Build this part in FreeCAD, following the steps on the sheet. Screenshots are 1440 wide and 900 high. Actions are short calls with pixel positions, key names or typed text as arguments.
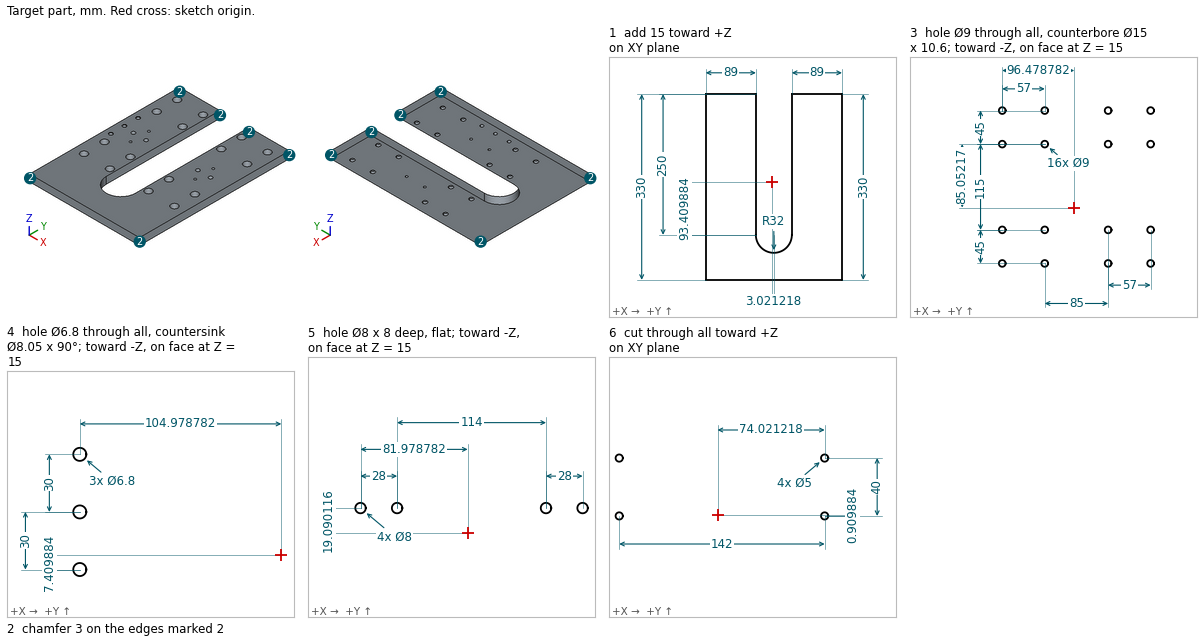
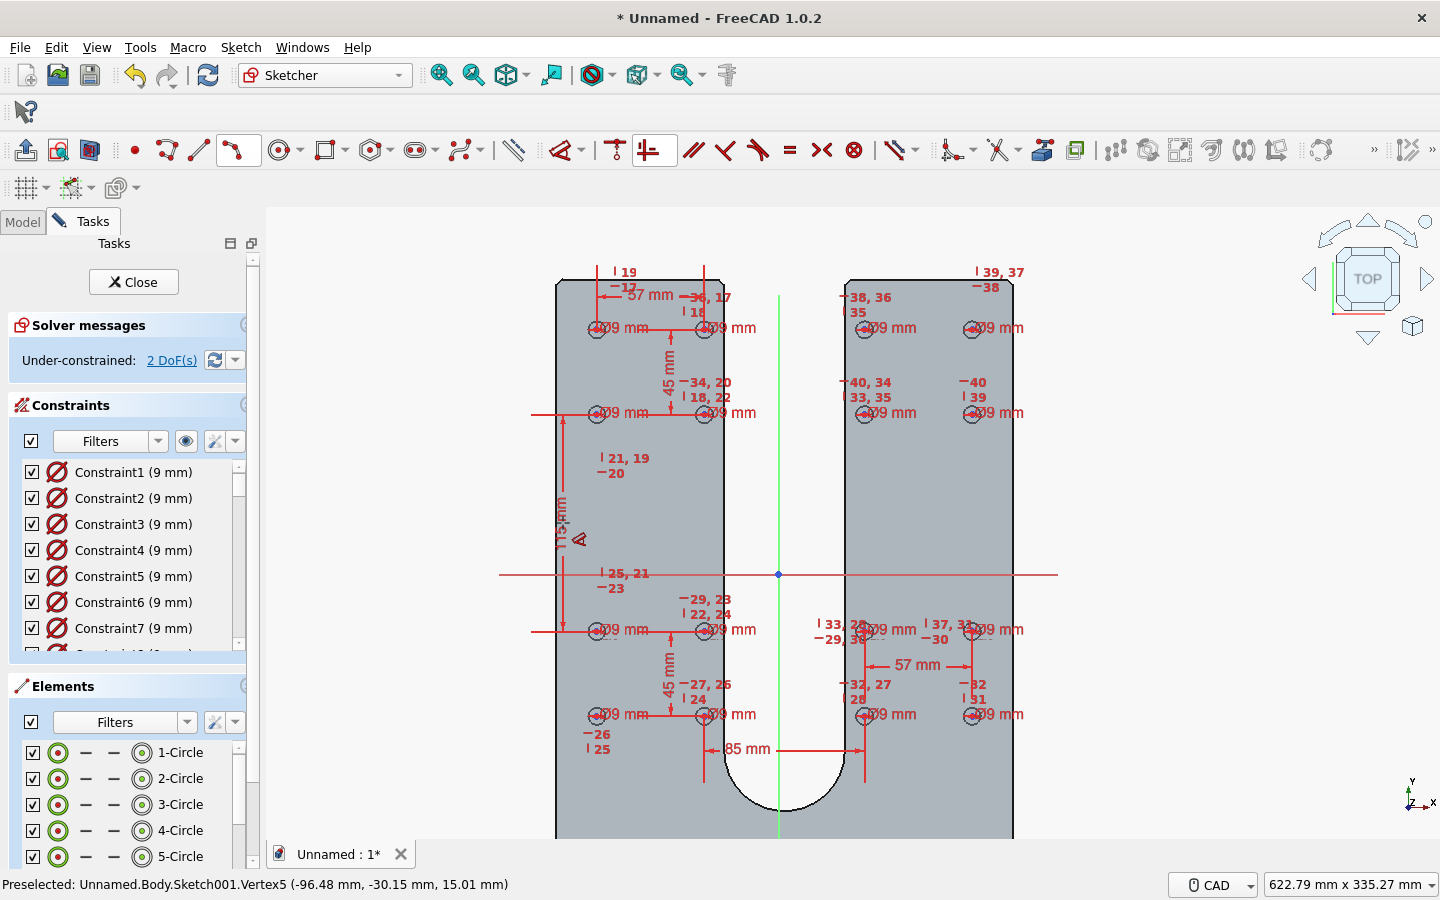
click(704, 415)
click(670, 495)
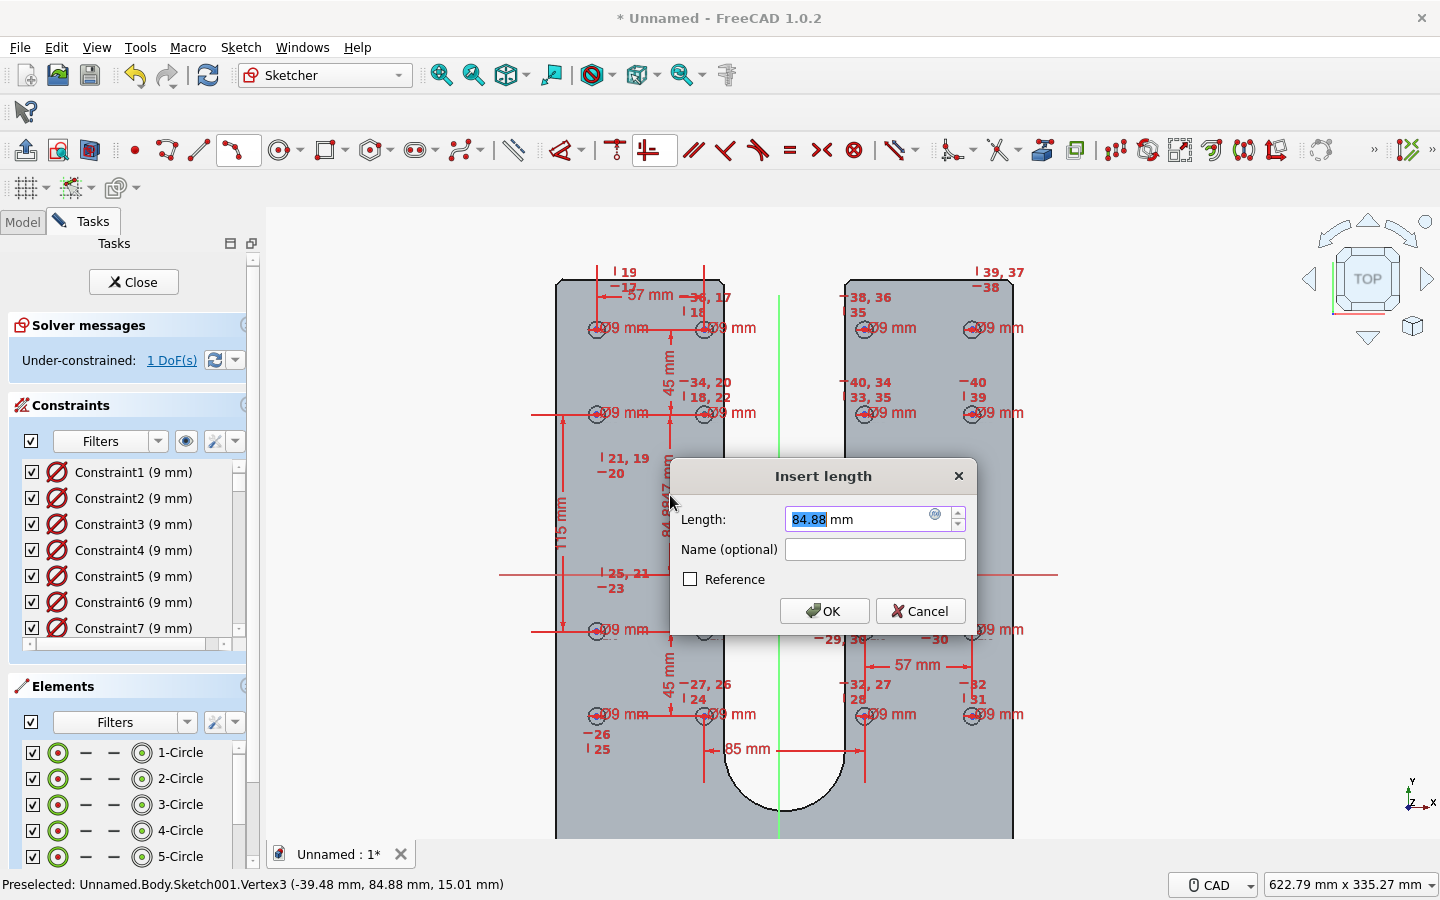
text(85.05217)
key(Return)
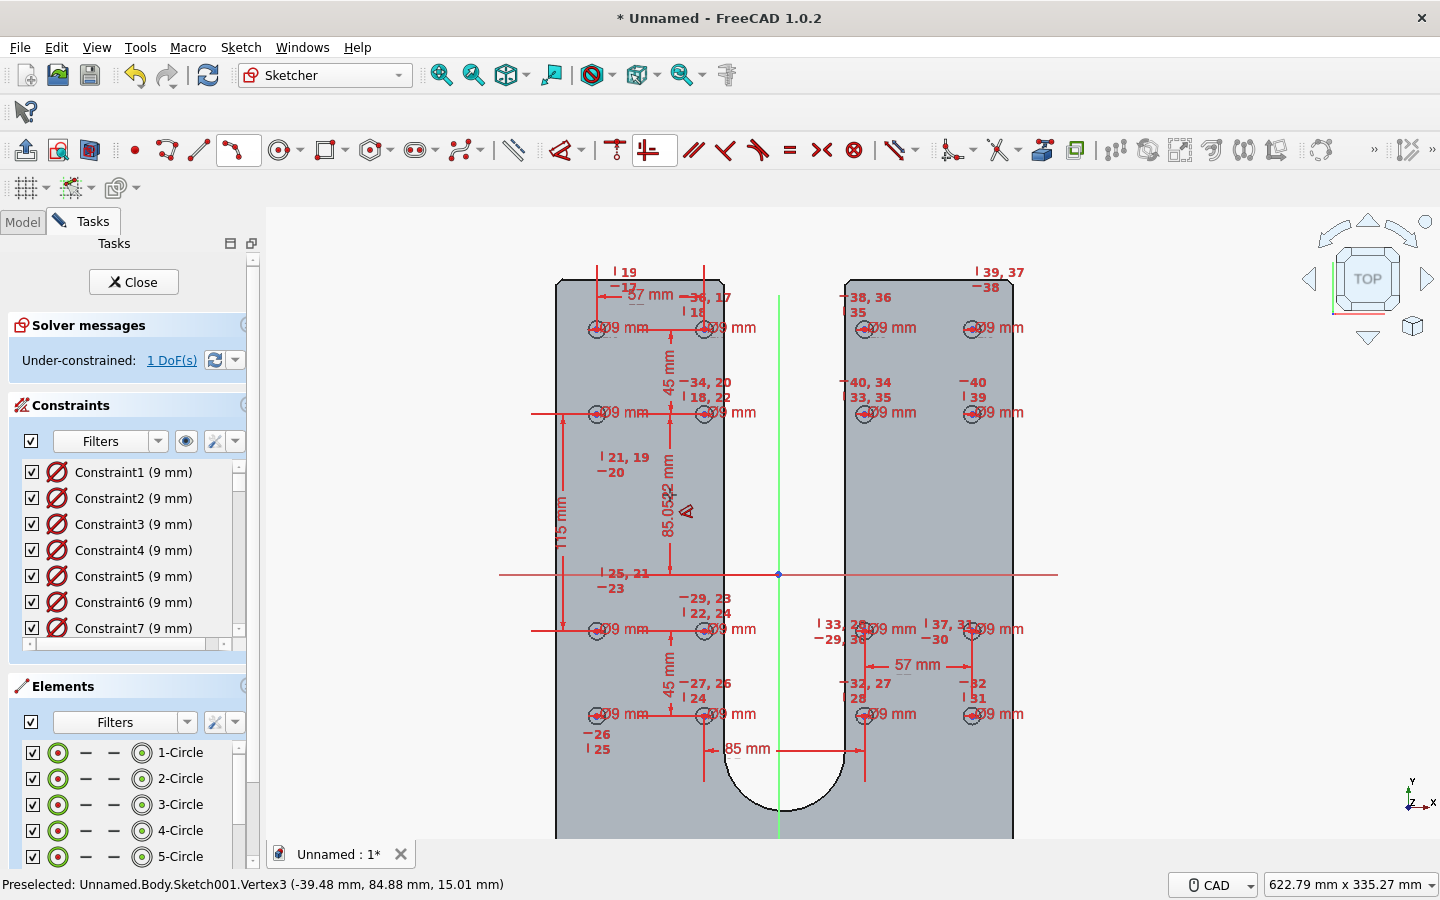
click(597, 330)
click(730, 296)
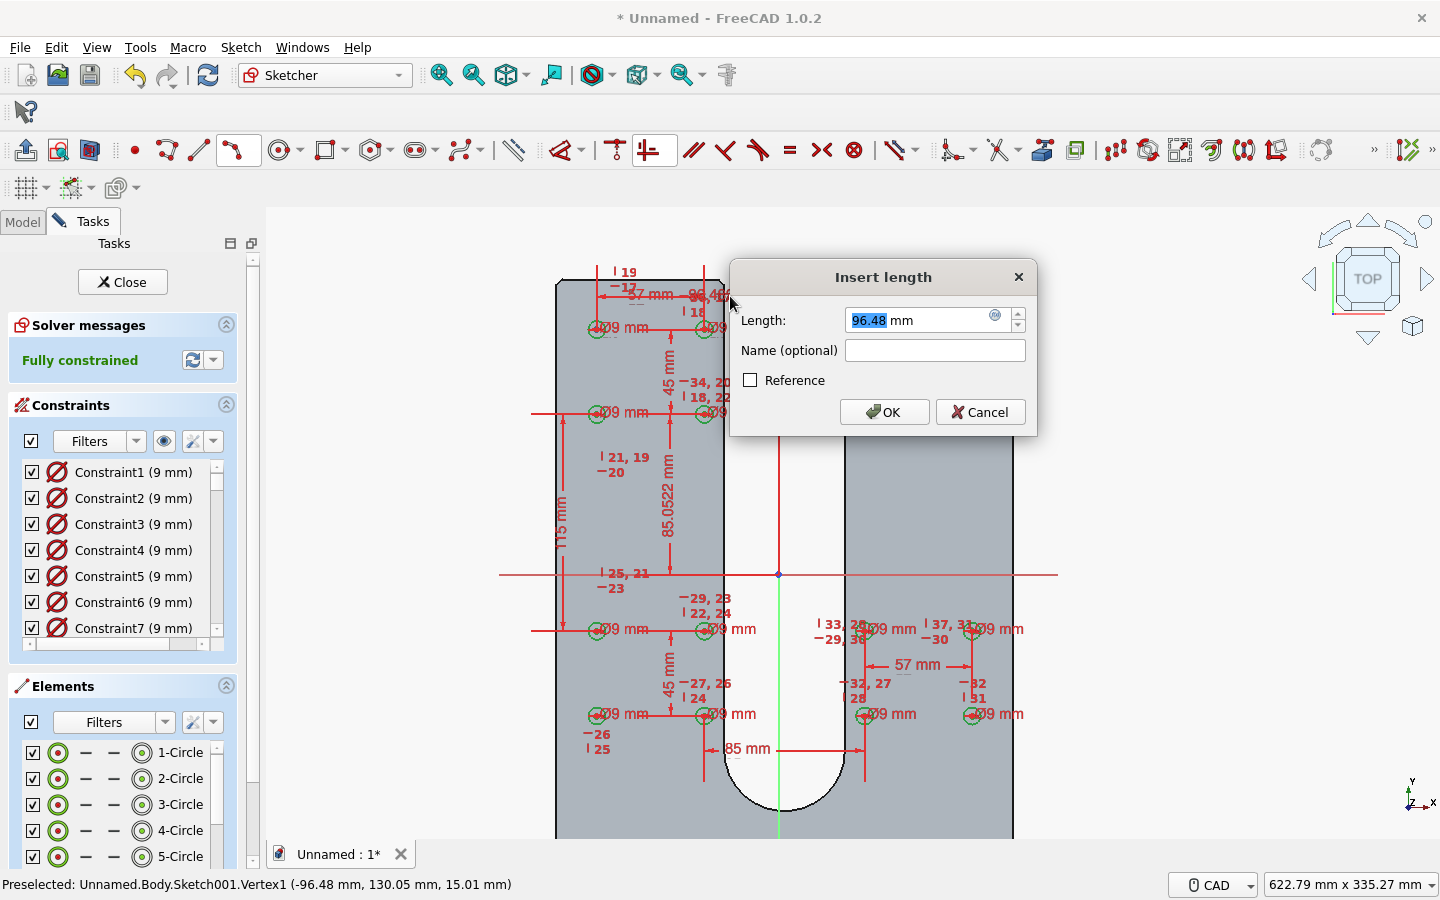
text(96.478782)
key(Return)
key(Escape)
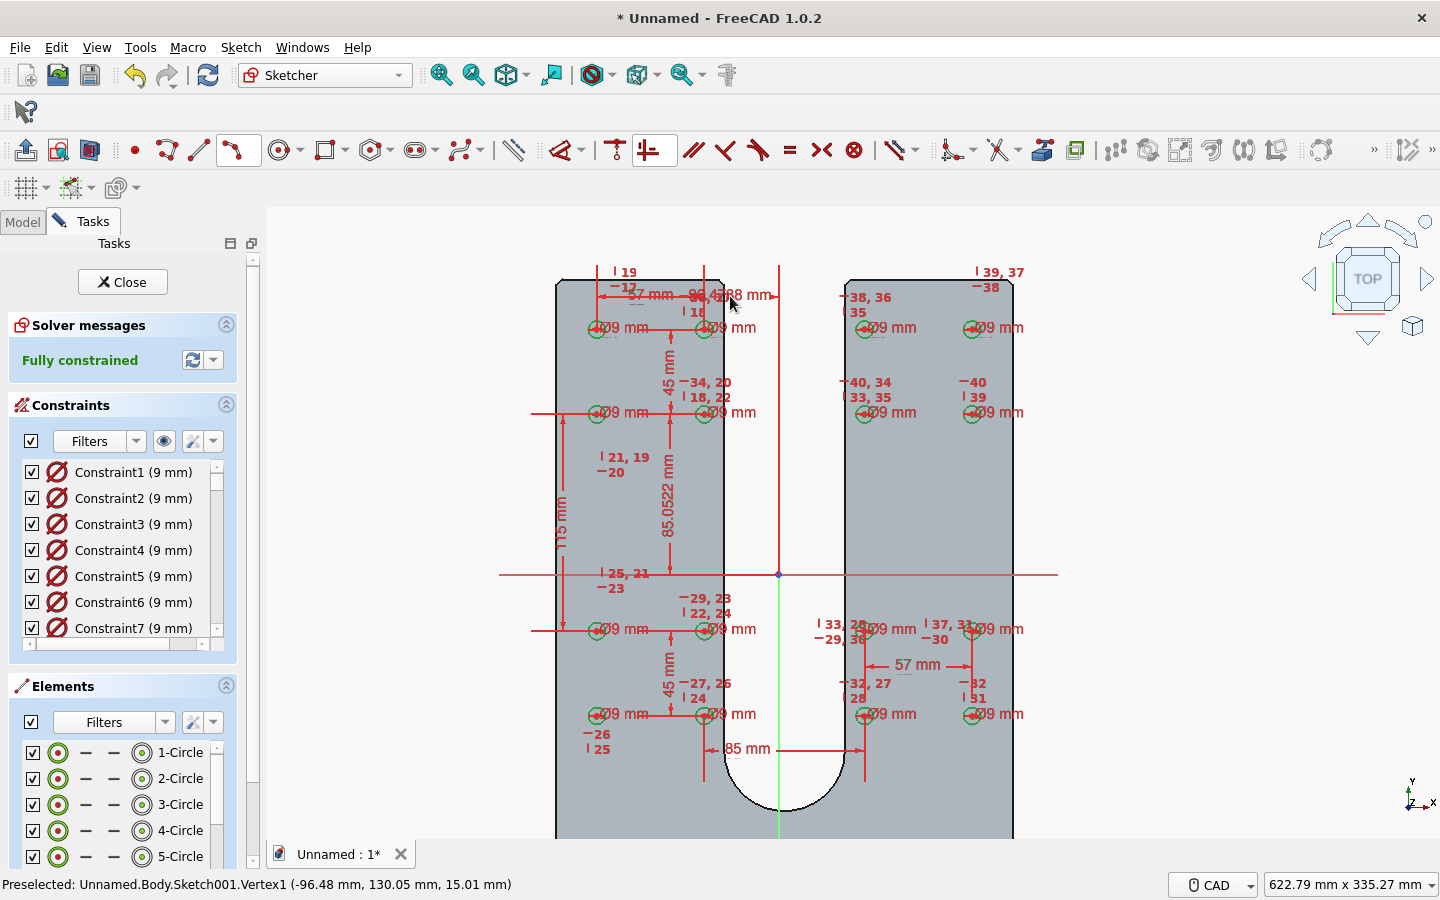
click(123, 282)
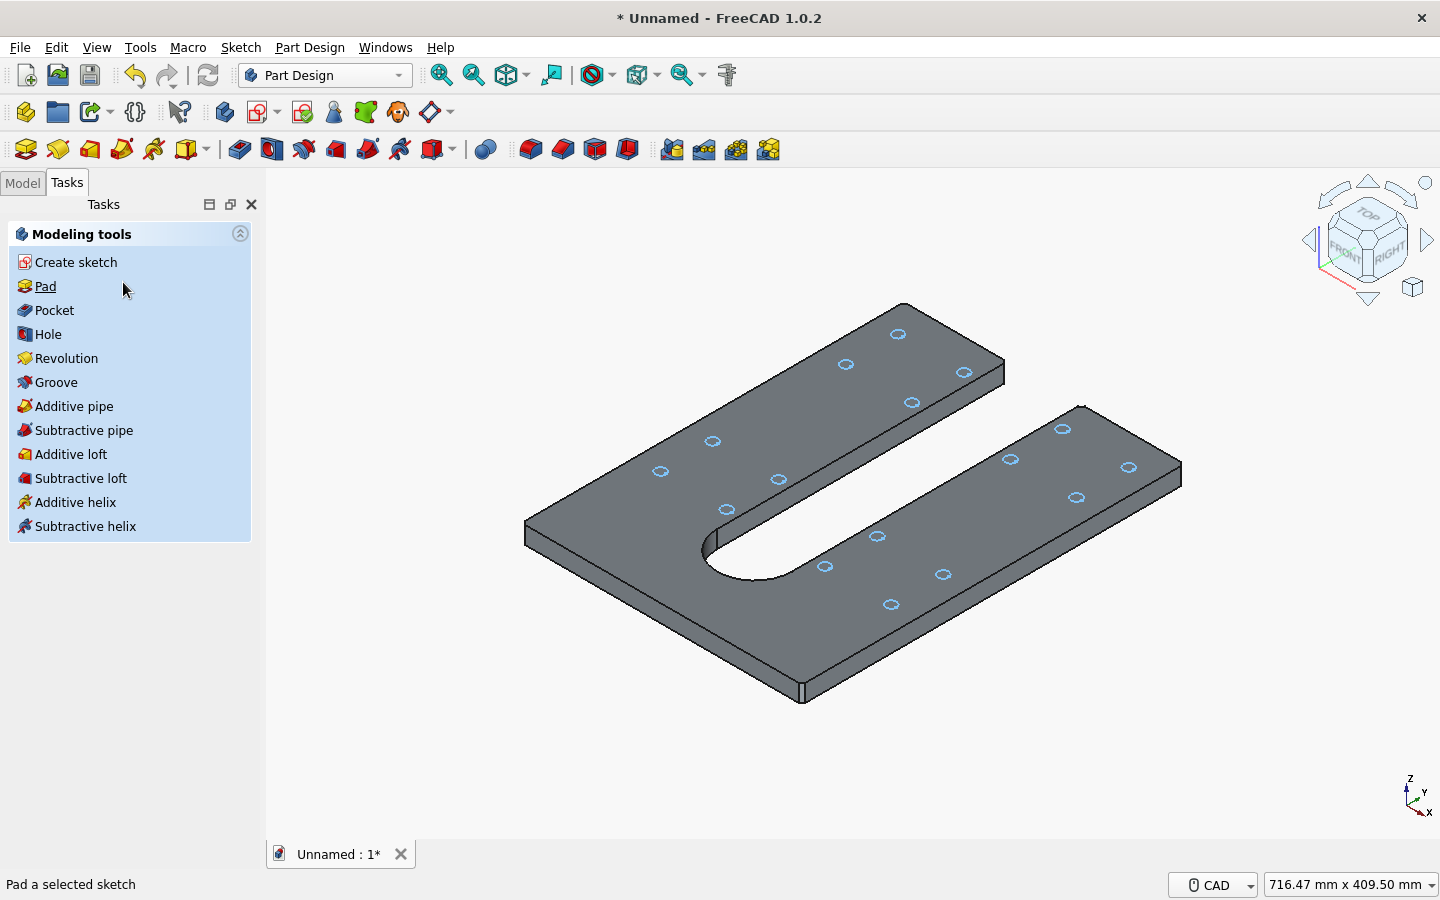
click(272, 150)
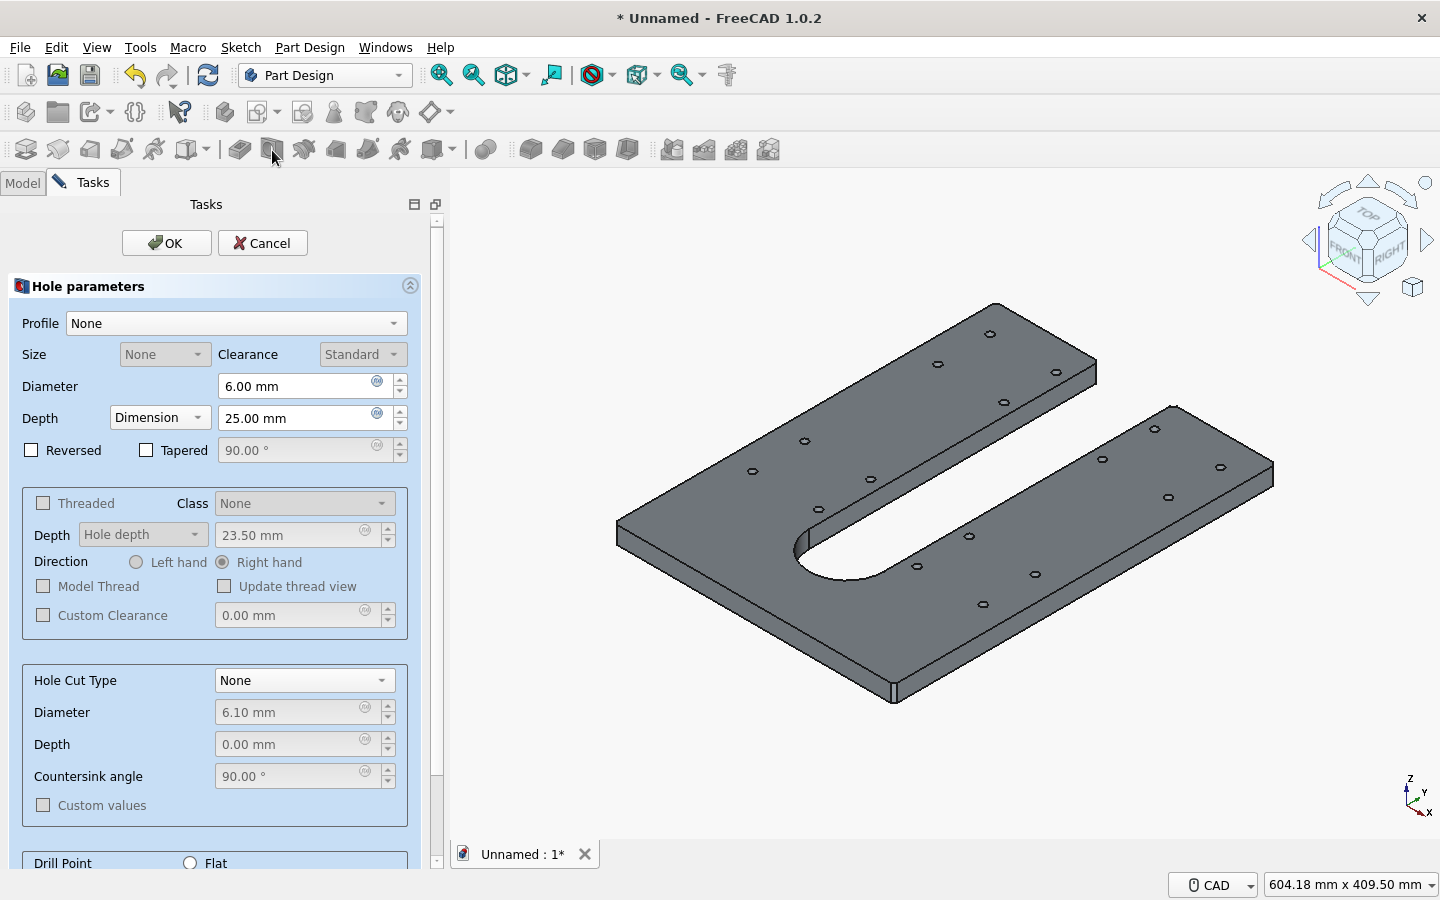
triple_click(305, 386)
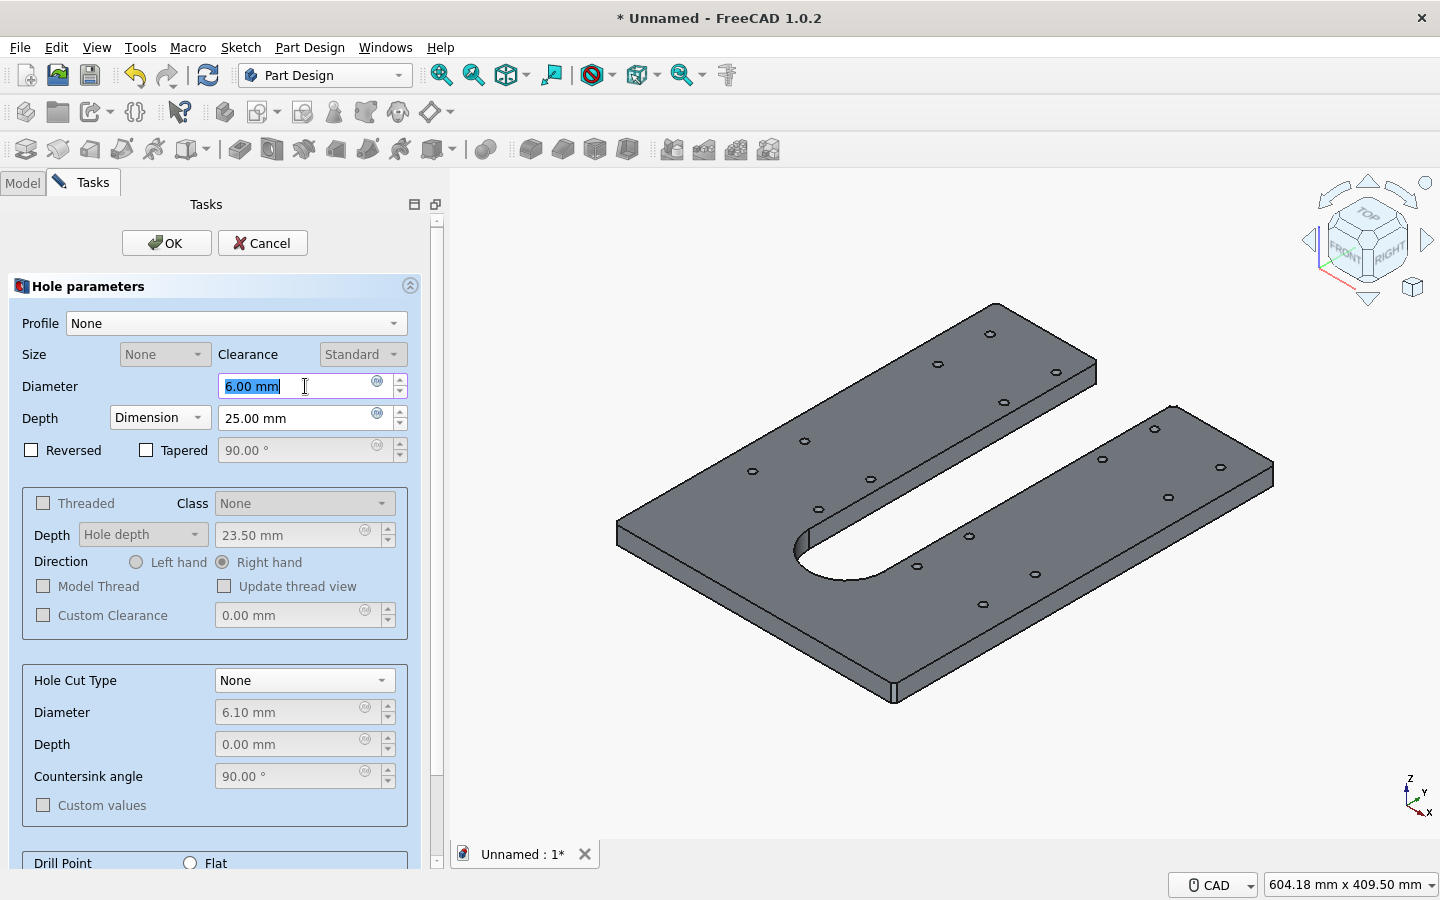
text(9)
key(Tab)